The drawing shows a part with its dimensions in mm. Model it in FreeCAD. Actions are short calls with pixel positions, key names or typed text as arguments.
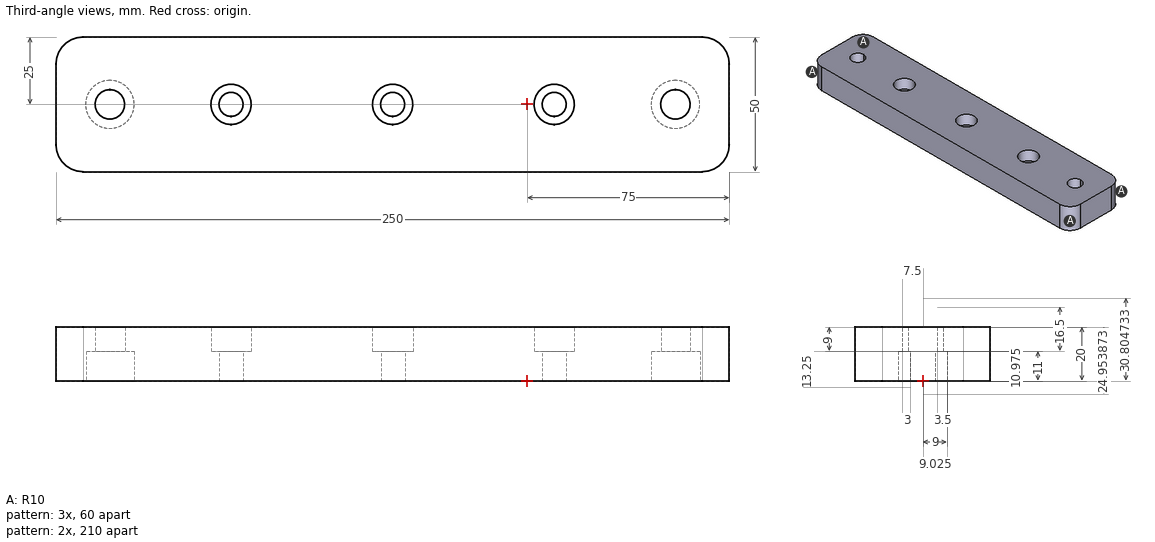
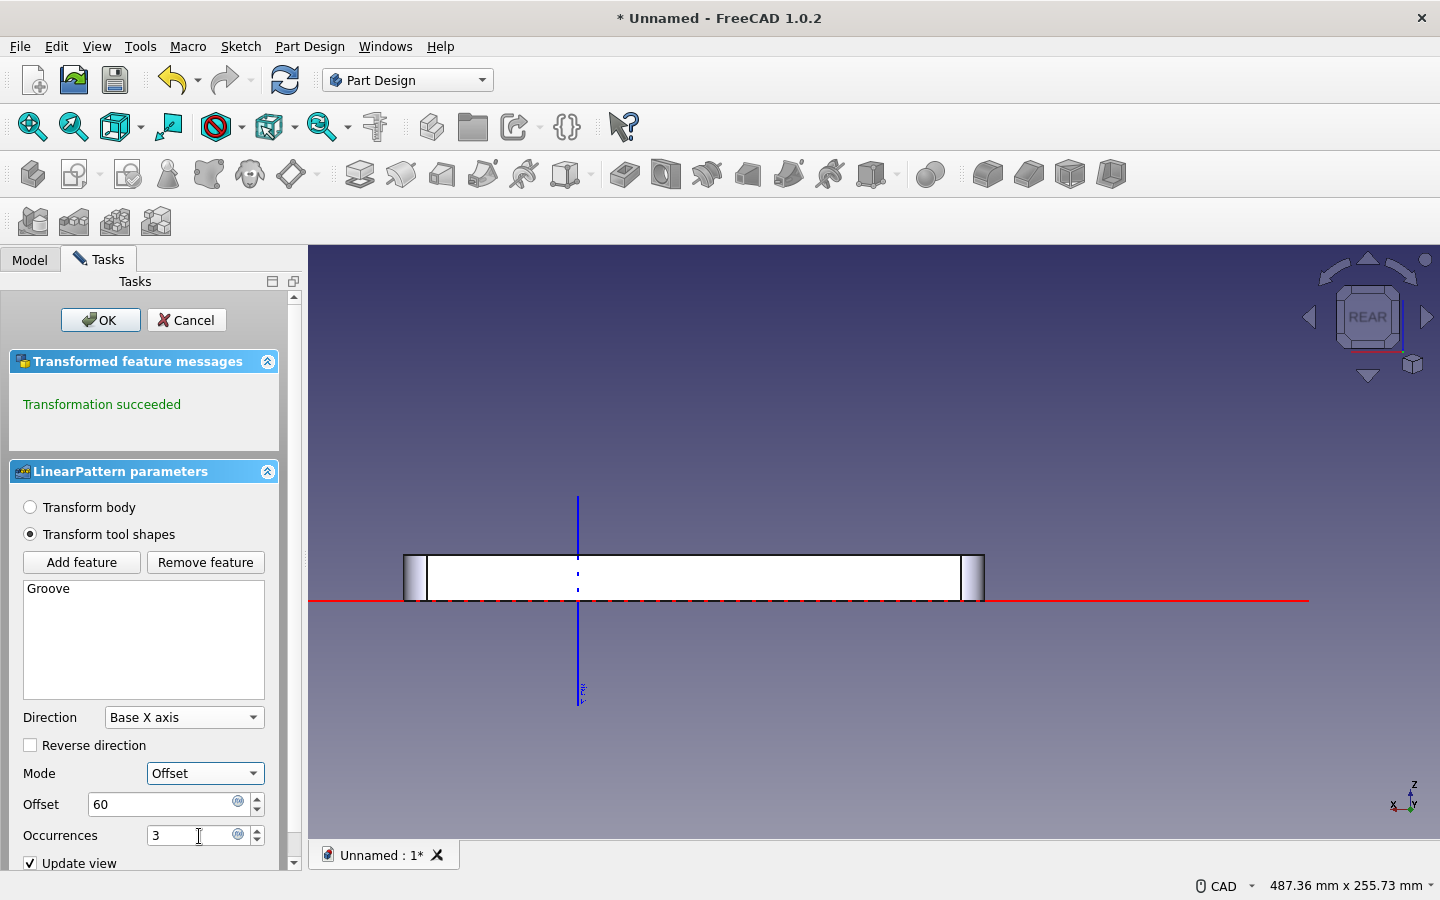
click(31, 745)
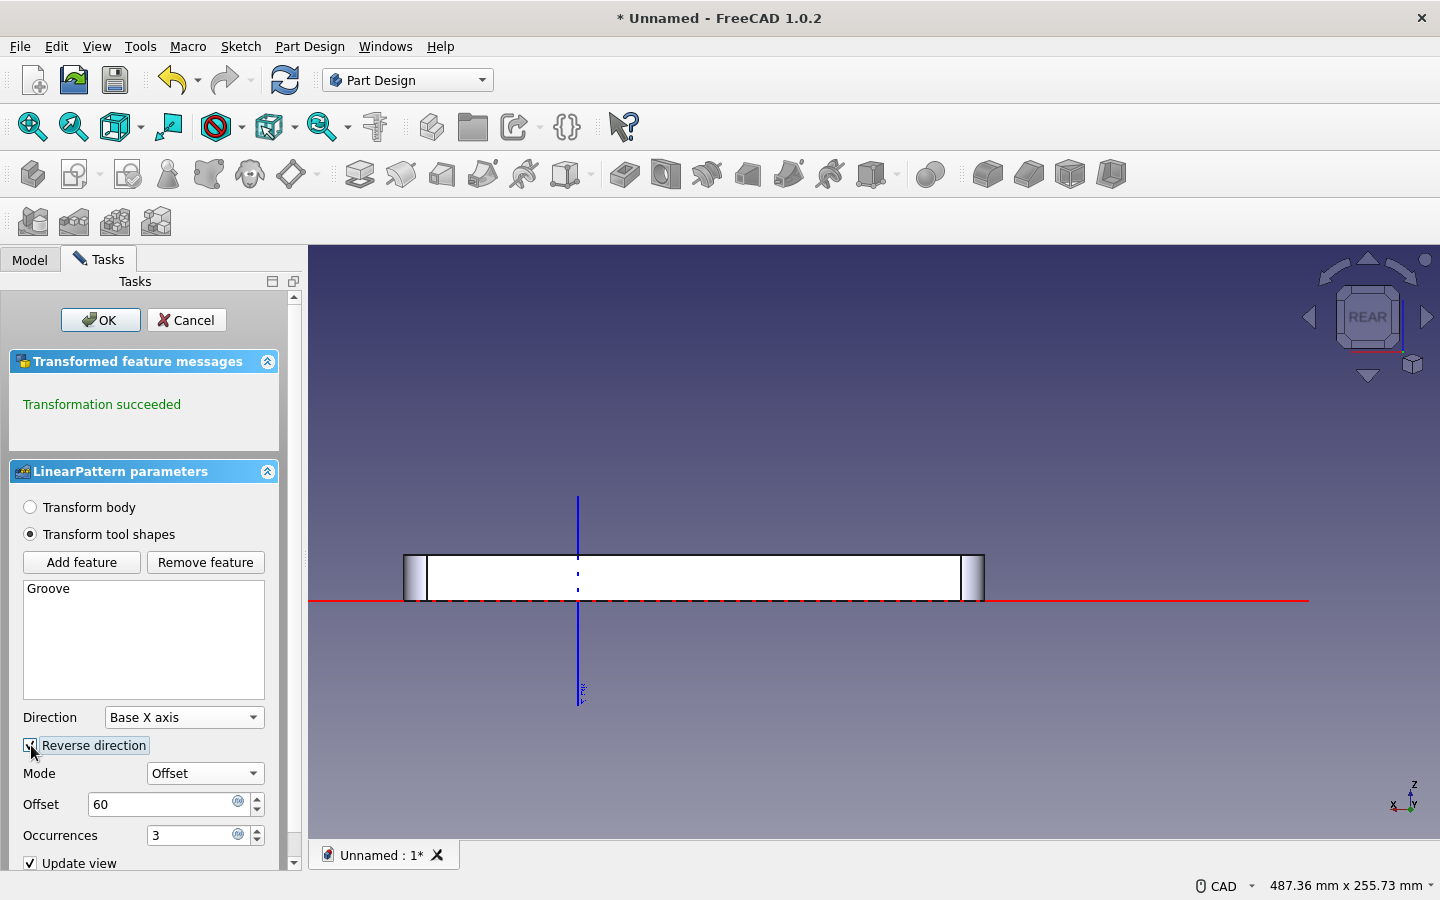
click(101, 320)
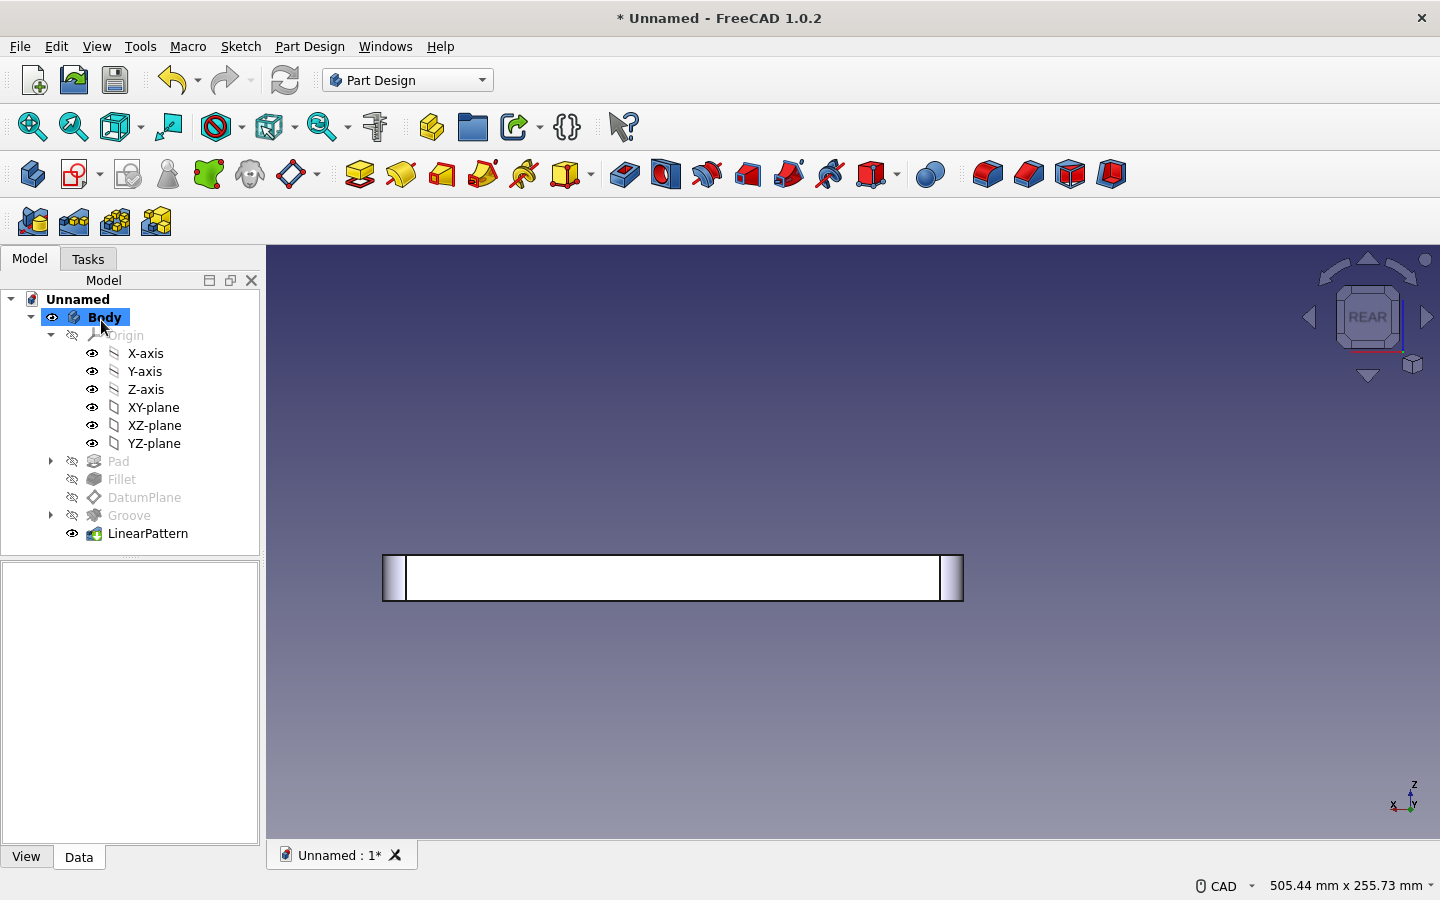
click(137, 443)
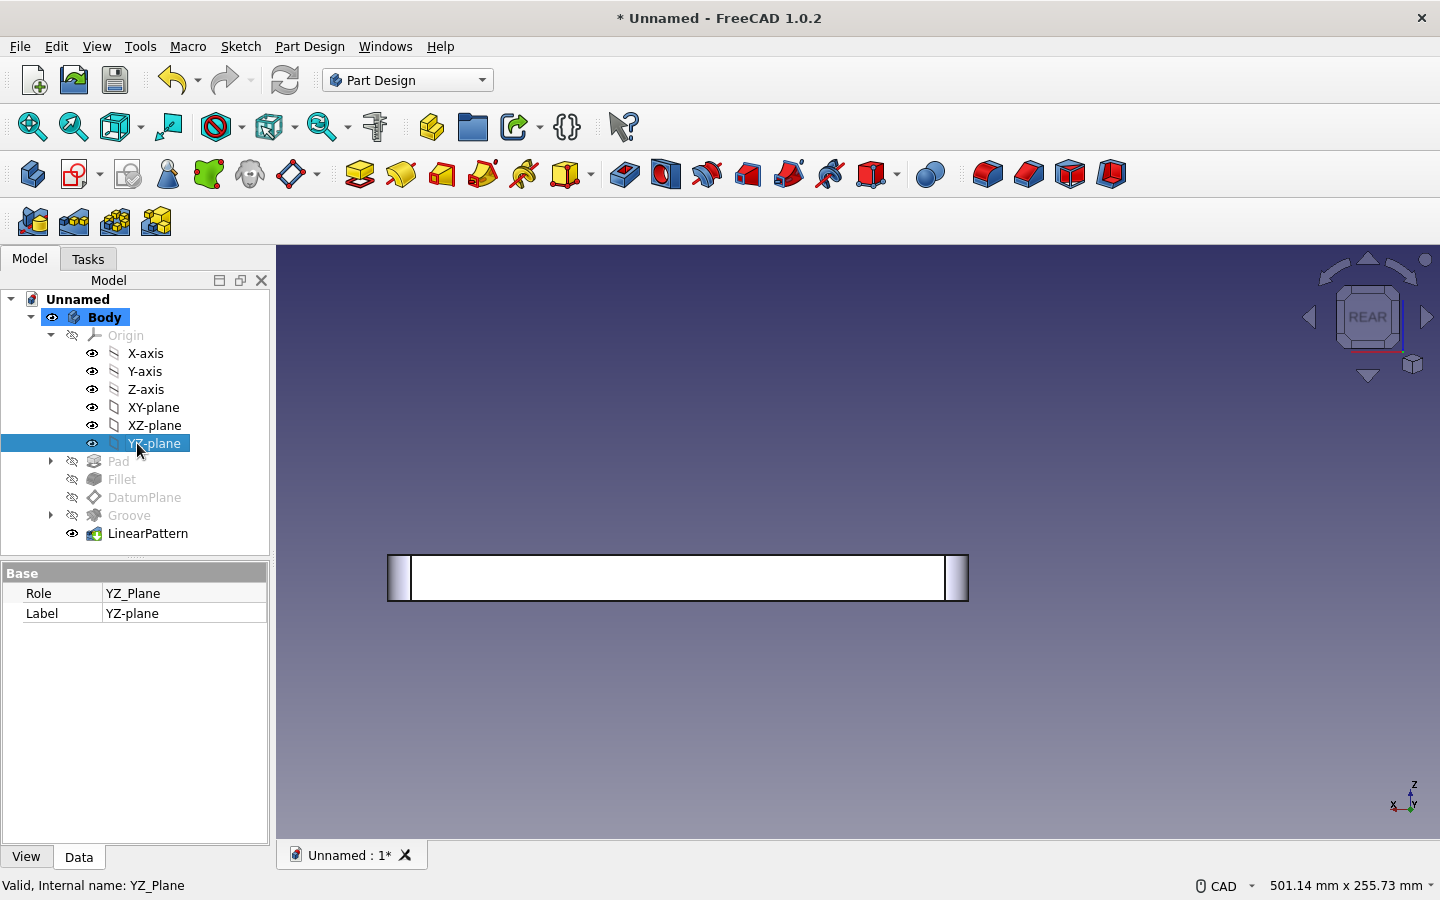
click(290, 174)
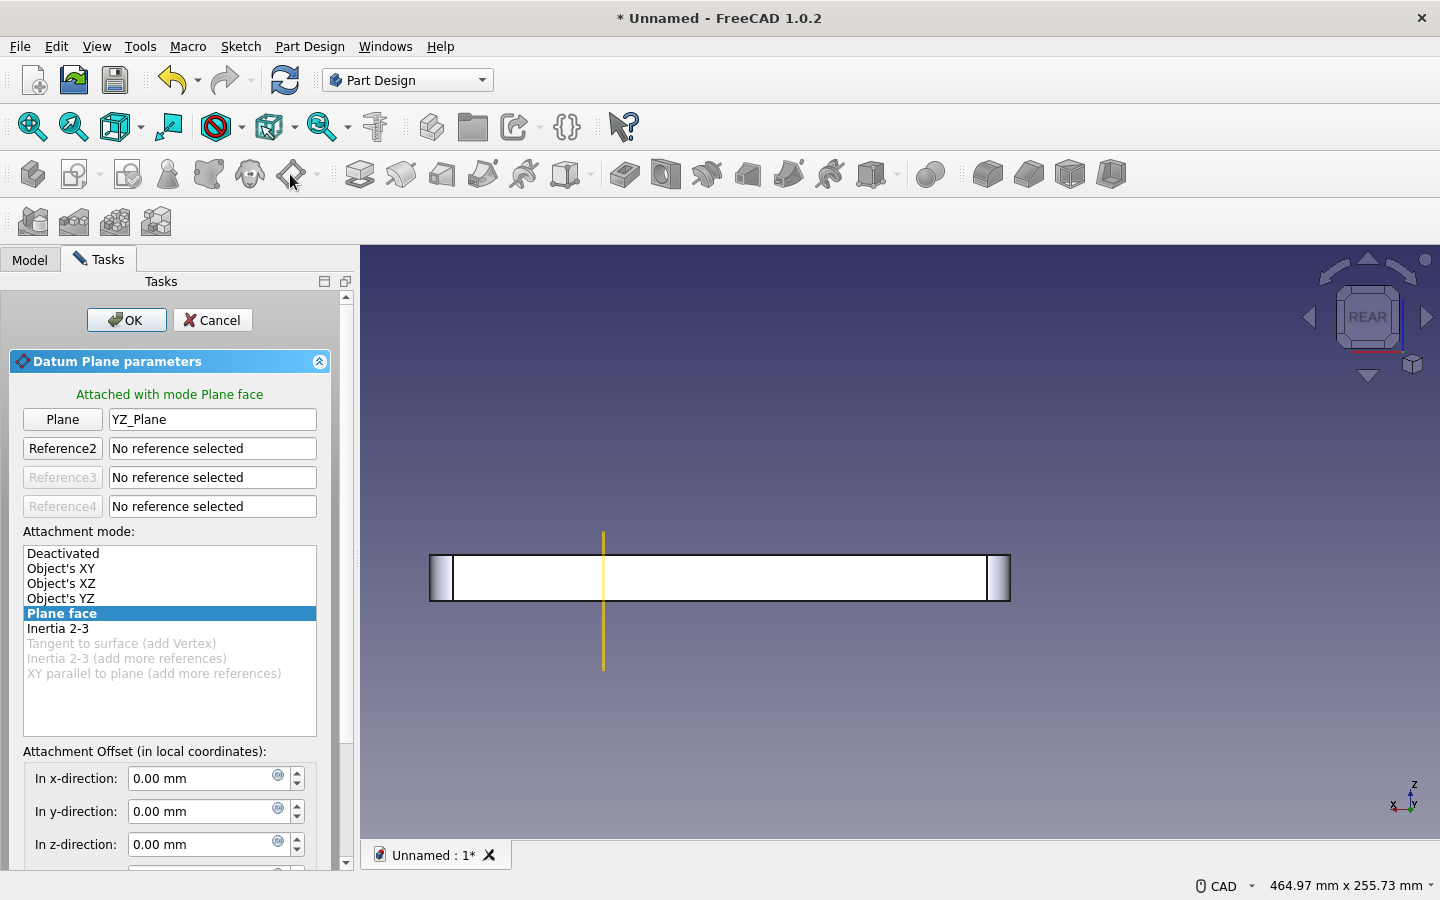
triple_click(210, 844)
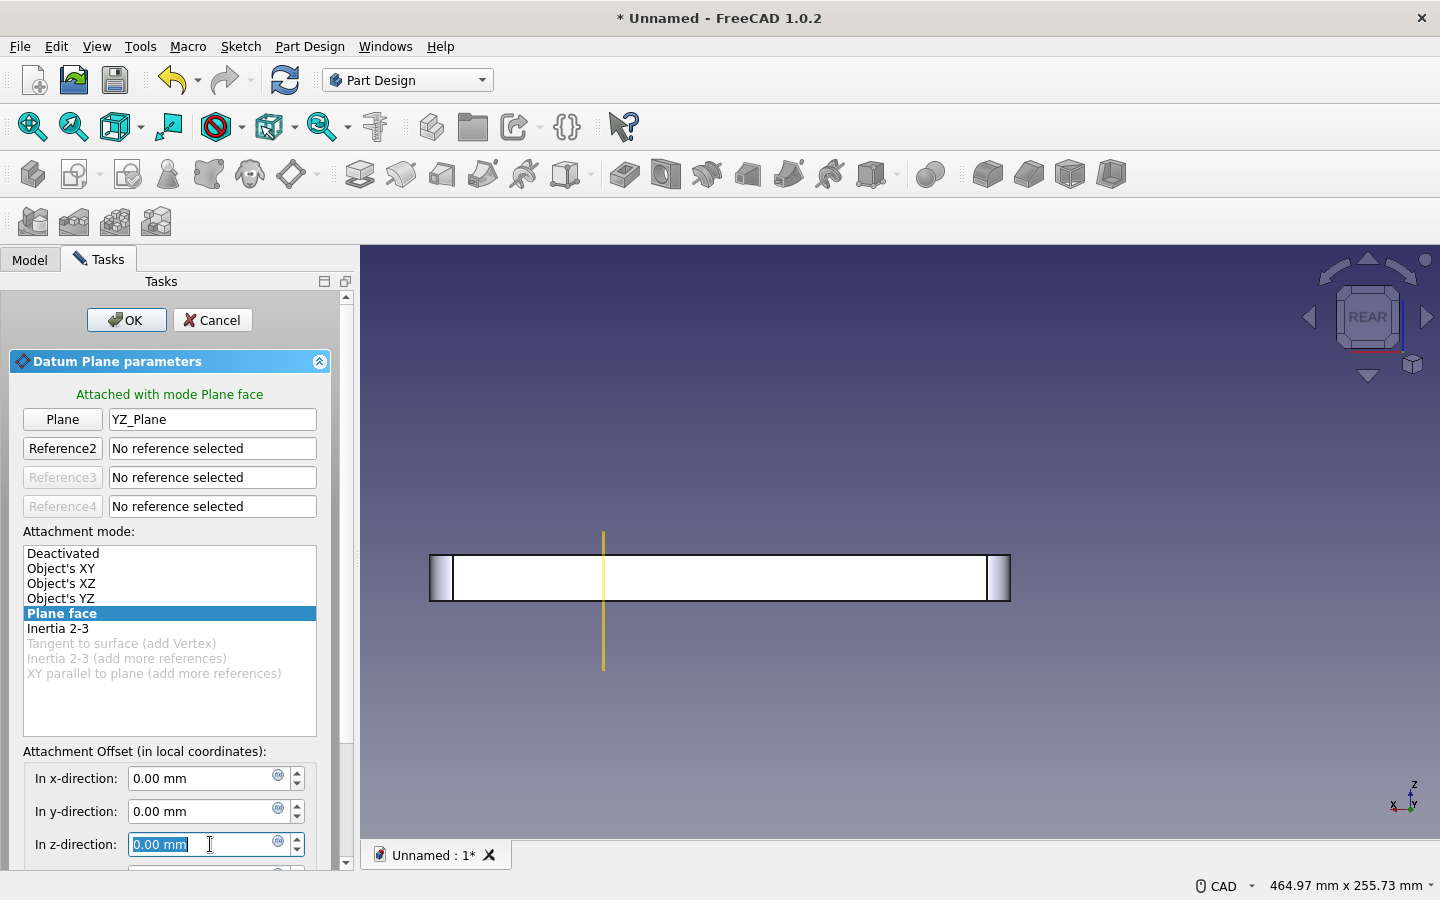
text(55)
key(Tab)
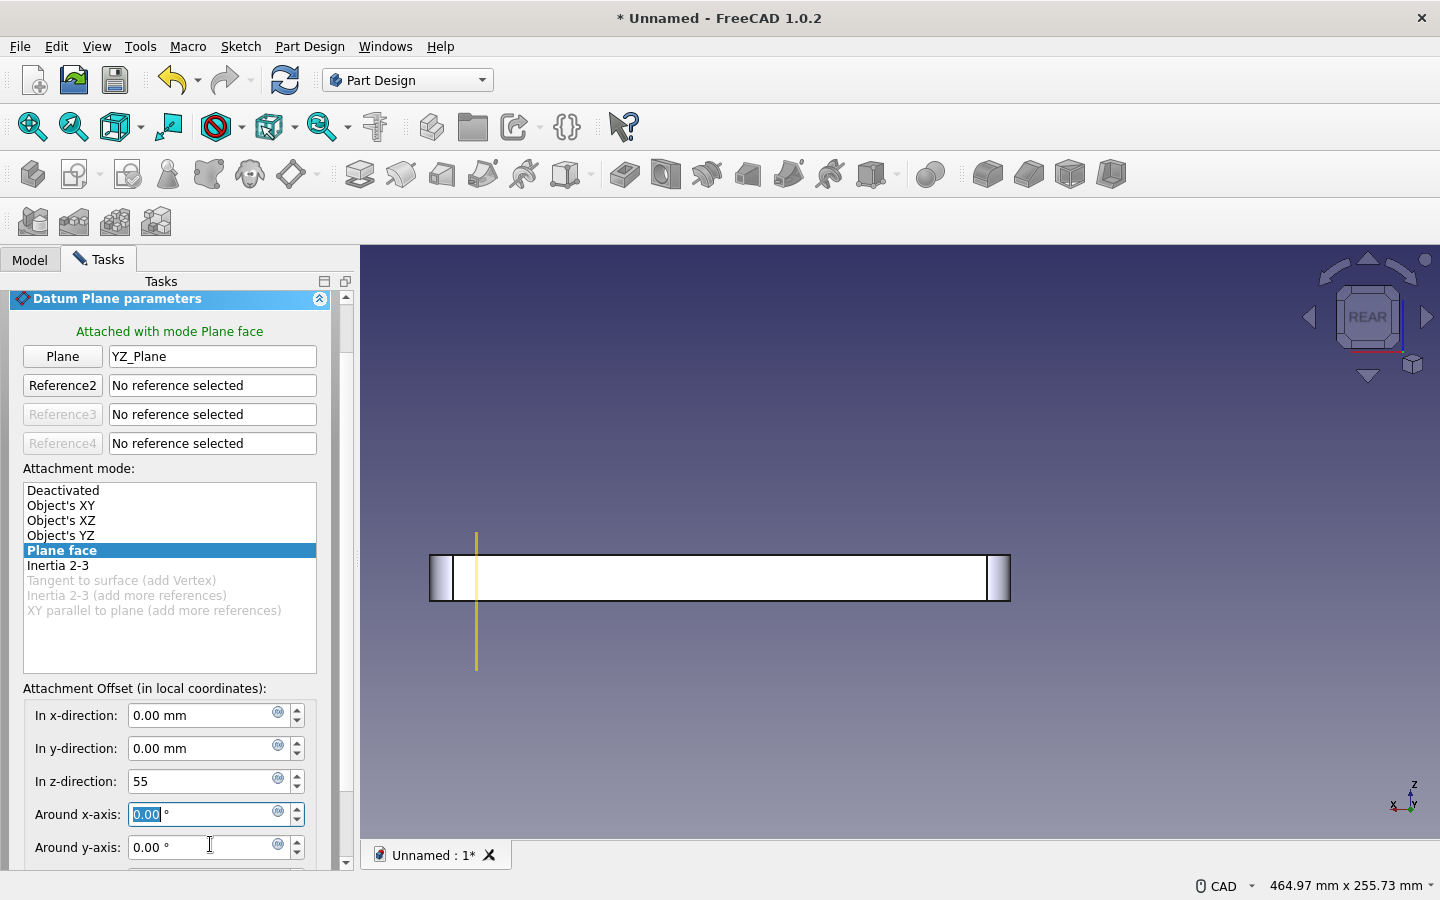
scroll(346, 580, up, 2)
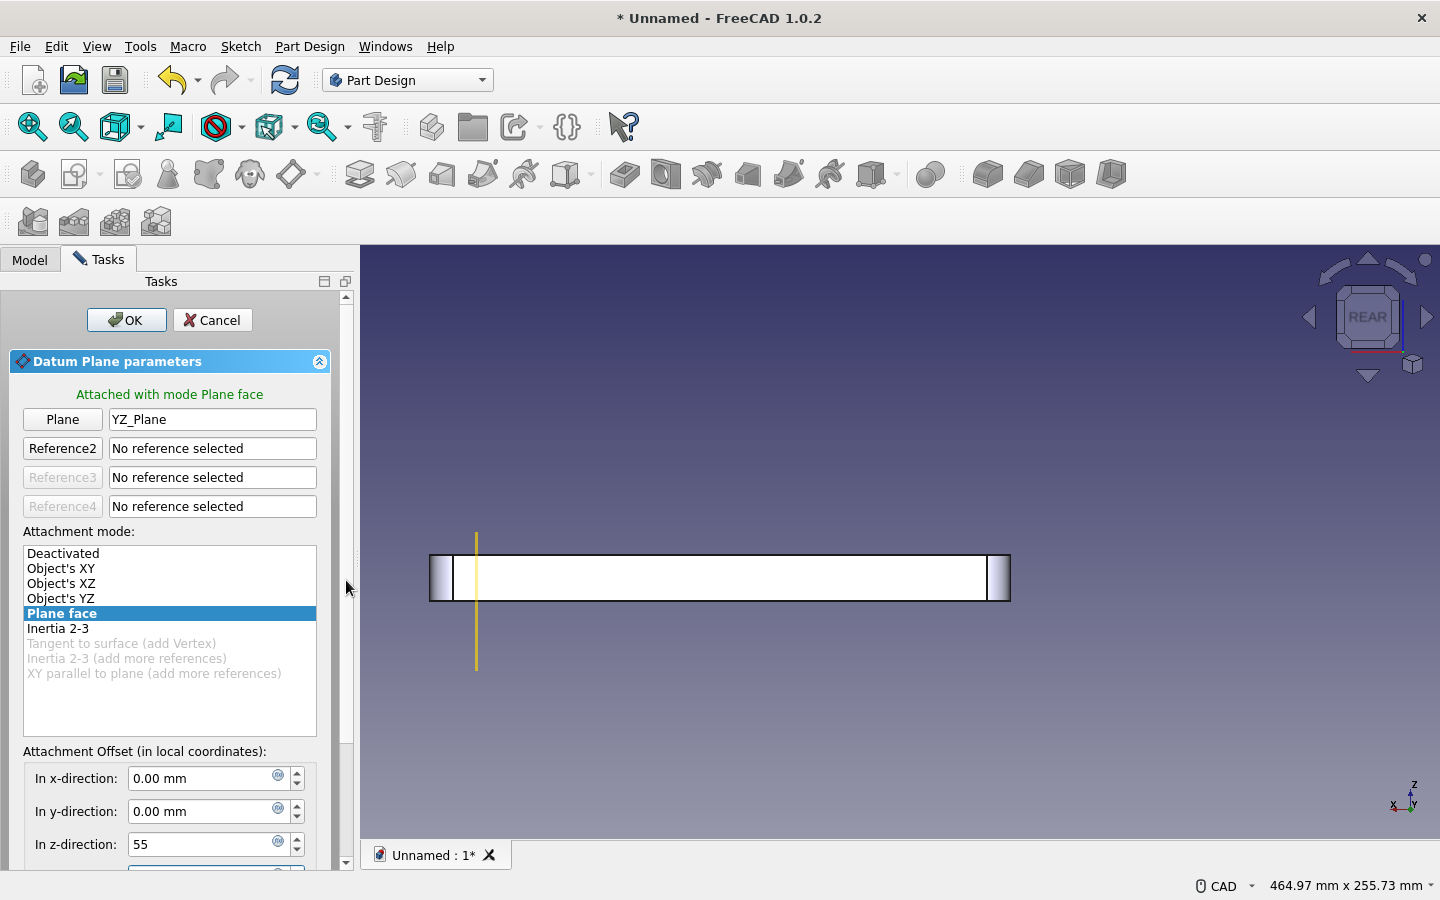
click(127, 320)